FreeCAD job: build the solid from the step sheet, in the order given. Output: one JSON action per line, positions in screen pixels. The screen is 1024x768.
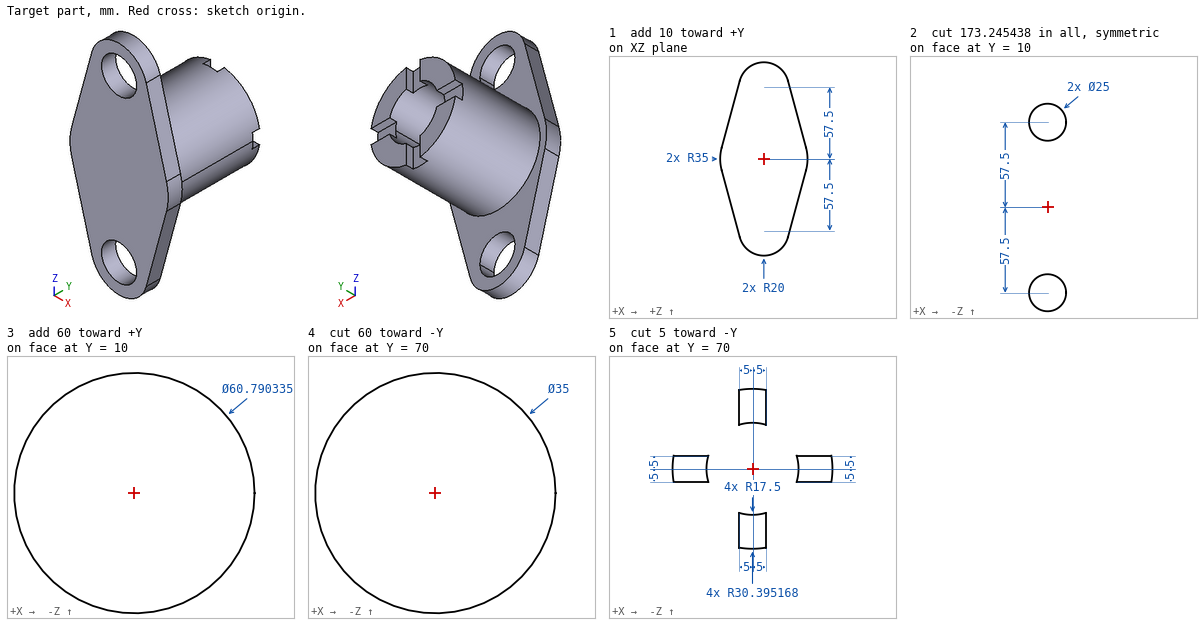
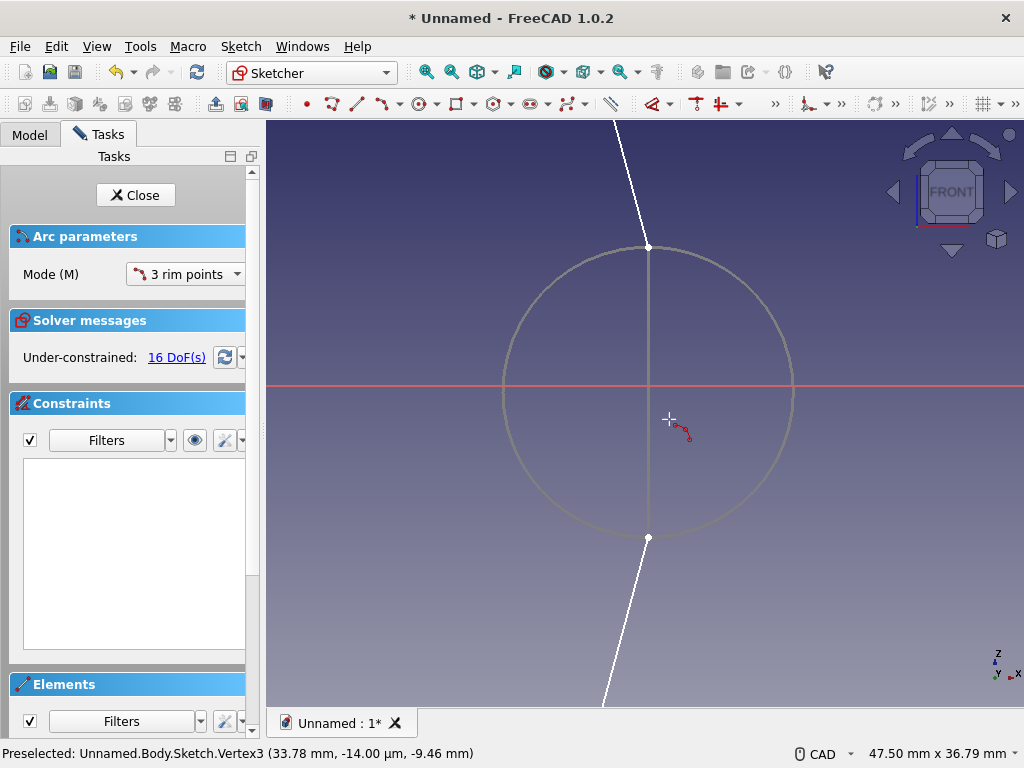
{"action": "left_click", "coordinate": [667, 416]}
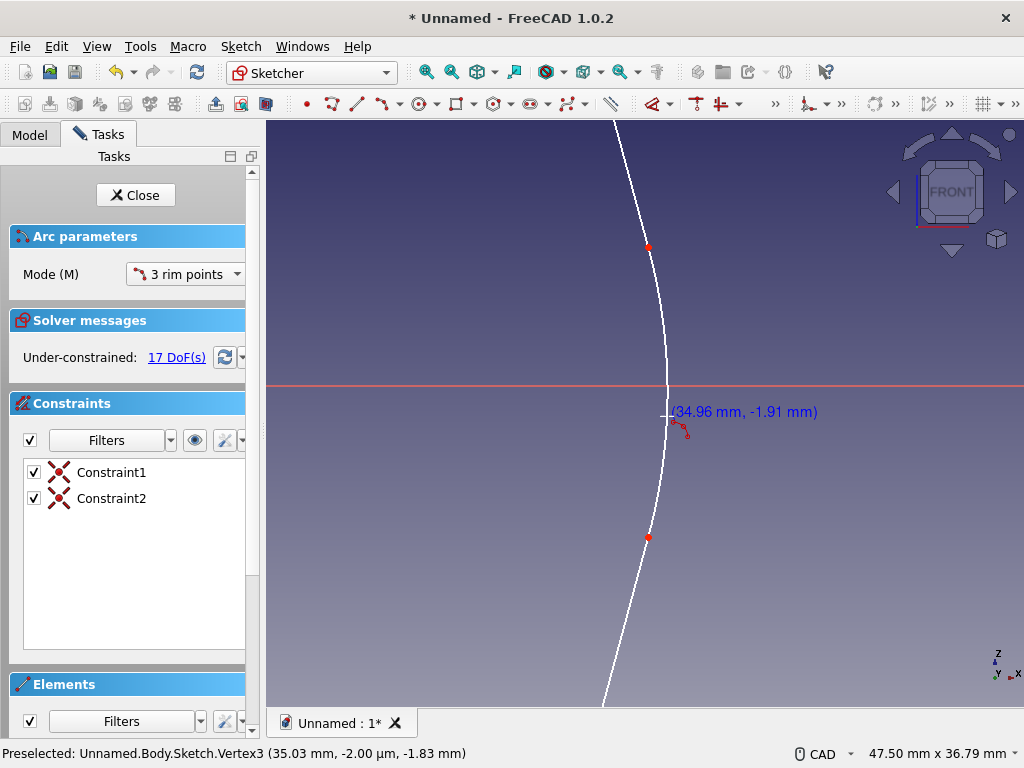
{"action": "scroll", "coordinate": [669, 419], "scroll_direction": "down", "scroll_amount": 9}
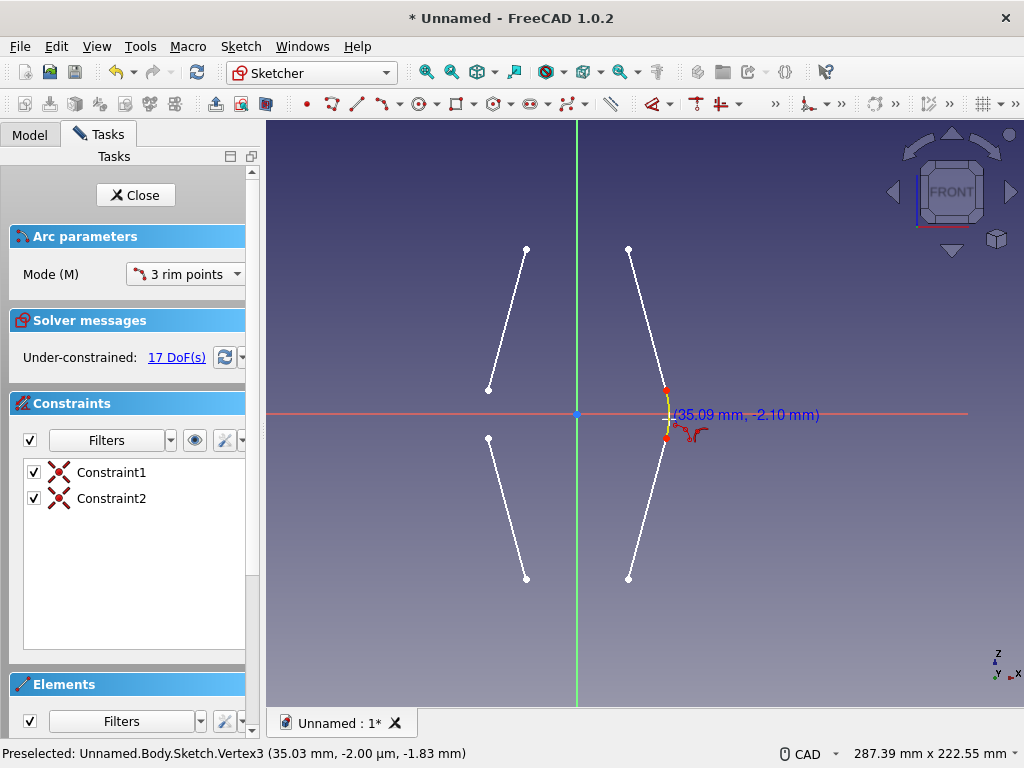
{"action": "left_click", "coordinate": [628, 580]}
{"action": "left_click", "coordinate": [526, 580]}
{"action": "left_click", "coordinate": [551, 611]}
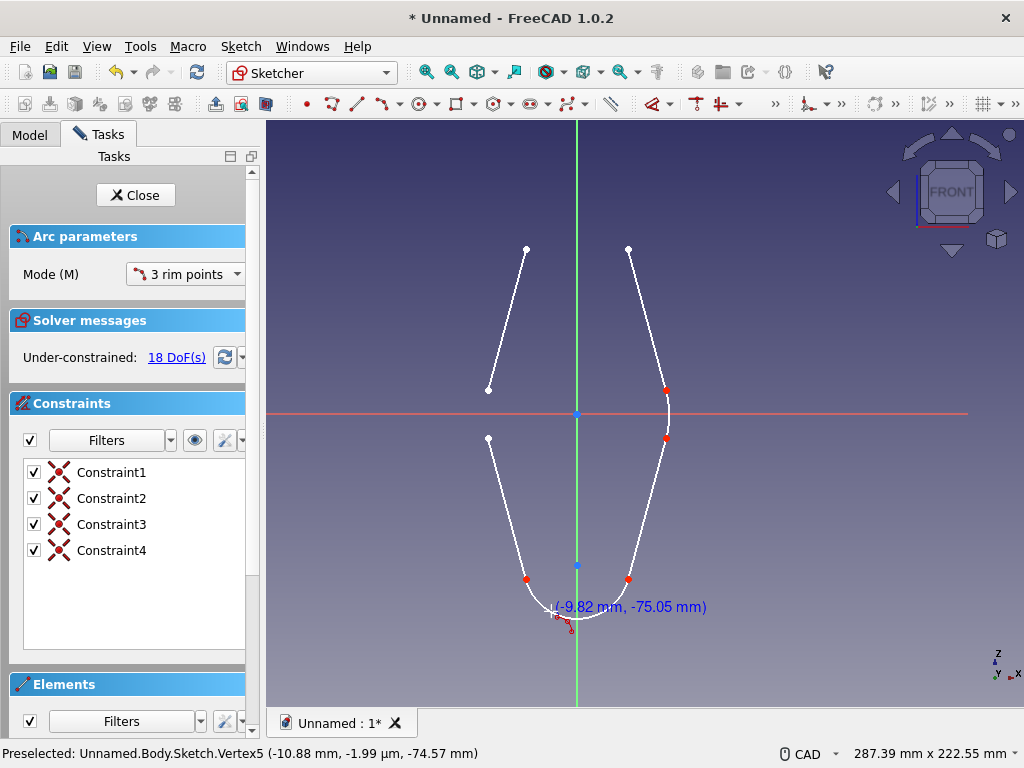
{"action": "left_click", "coordinate": [488, 439]}
{"action": "left_click", "coordinate": [488, 391]}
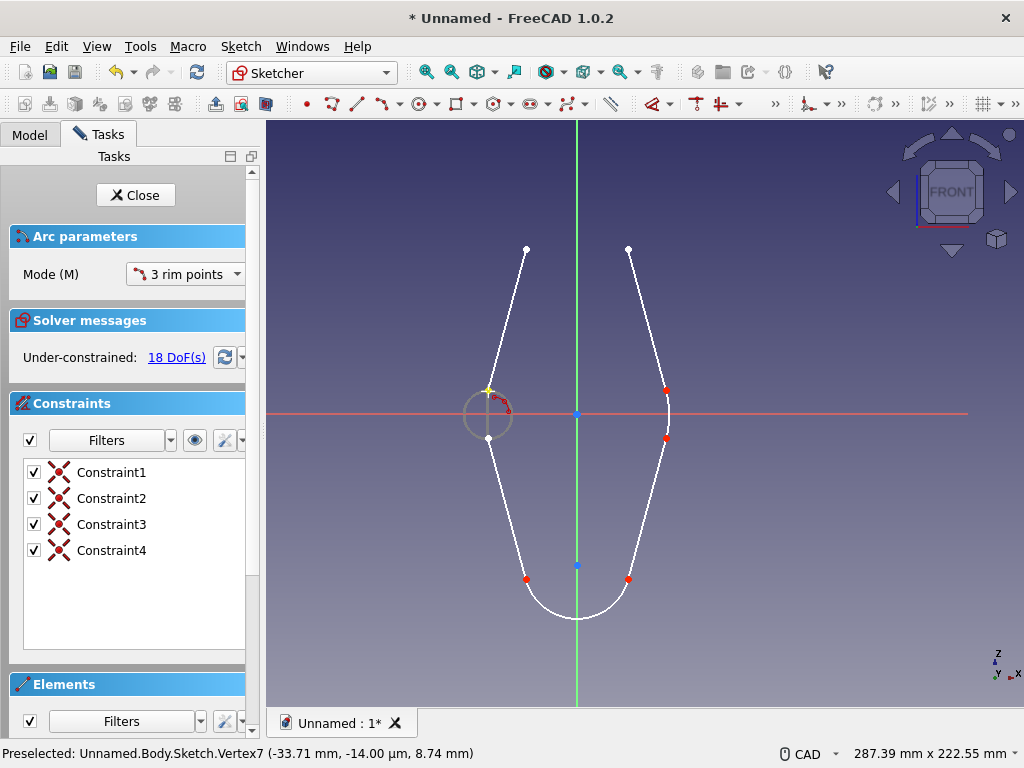
{"action": "scroll", "coordinate": [485, 409], "scroll_direction": "up", "scroll_amount": 9}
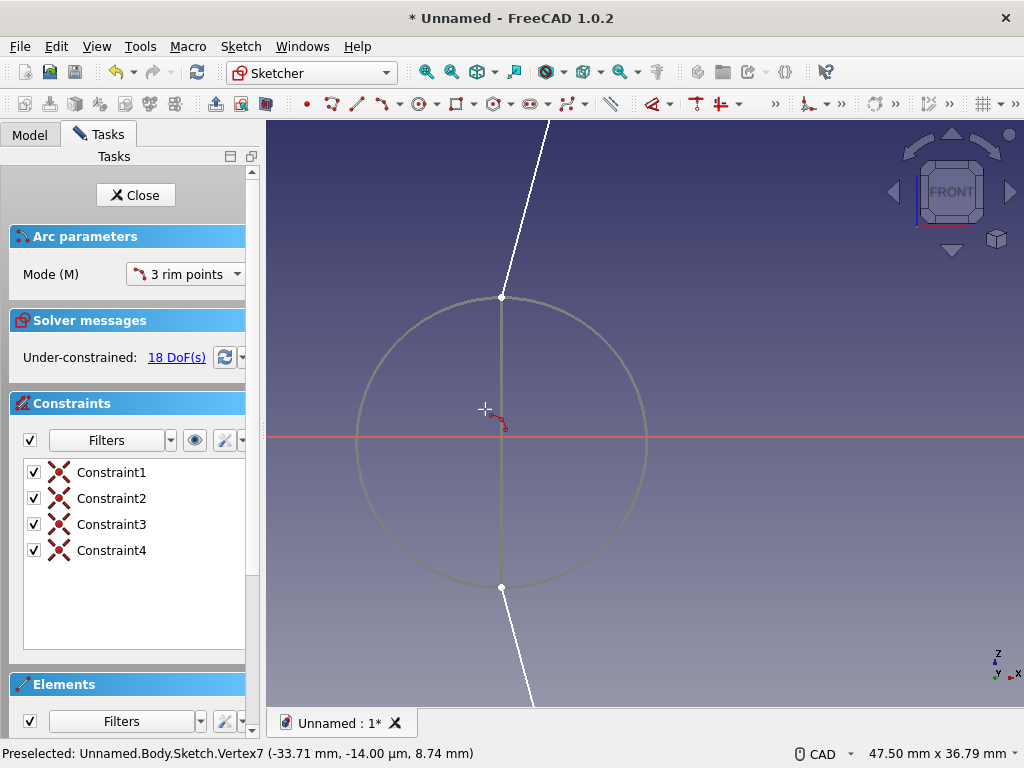
{"action": "left_click", "coordinate": [482, 408]}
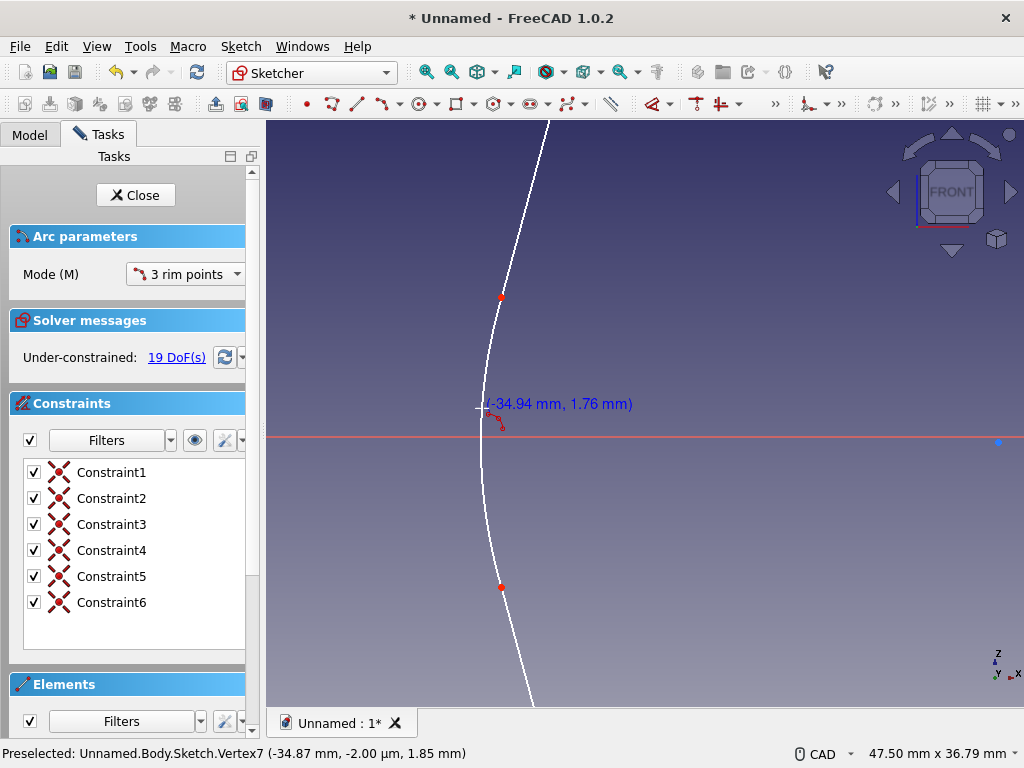
{"action": "scroll", "coordinate": [485, 409], "scroll_direction": "down", "scroll_amount": 9}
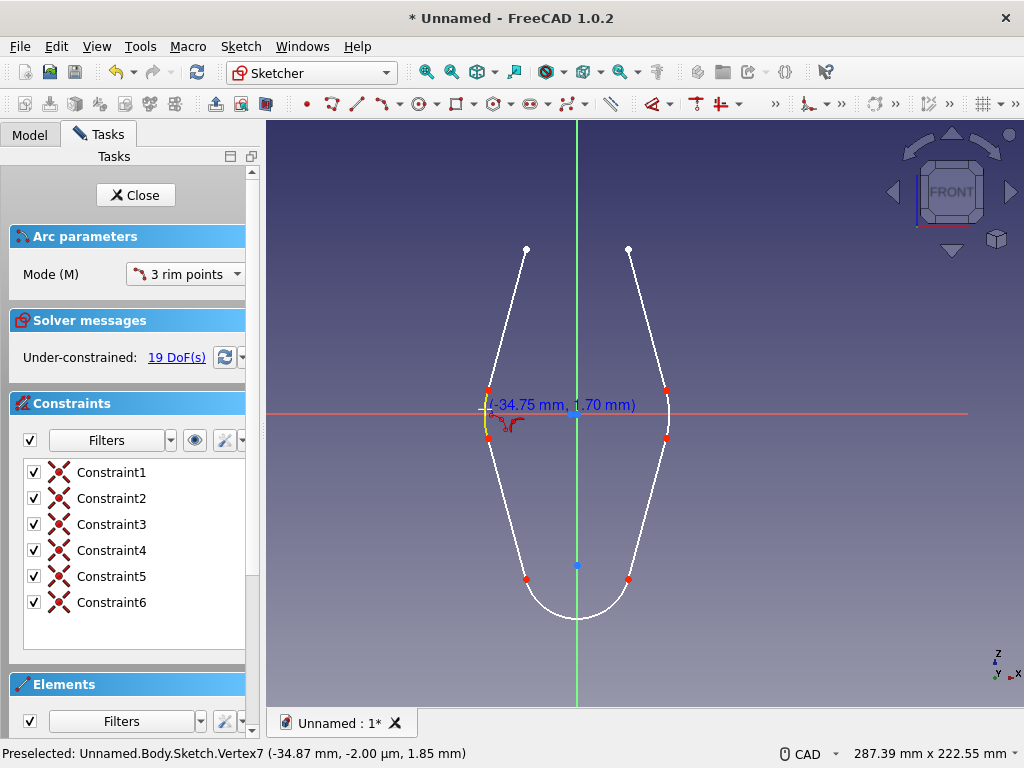
{"action": "left_click", "coordinate": [526, 250]}
{"action": "left_click", "coordinate": [628, 250]}
{"action": "left_click", "coordinate": [603, 217]}
{"action": "key", "text": "Escape"}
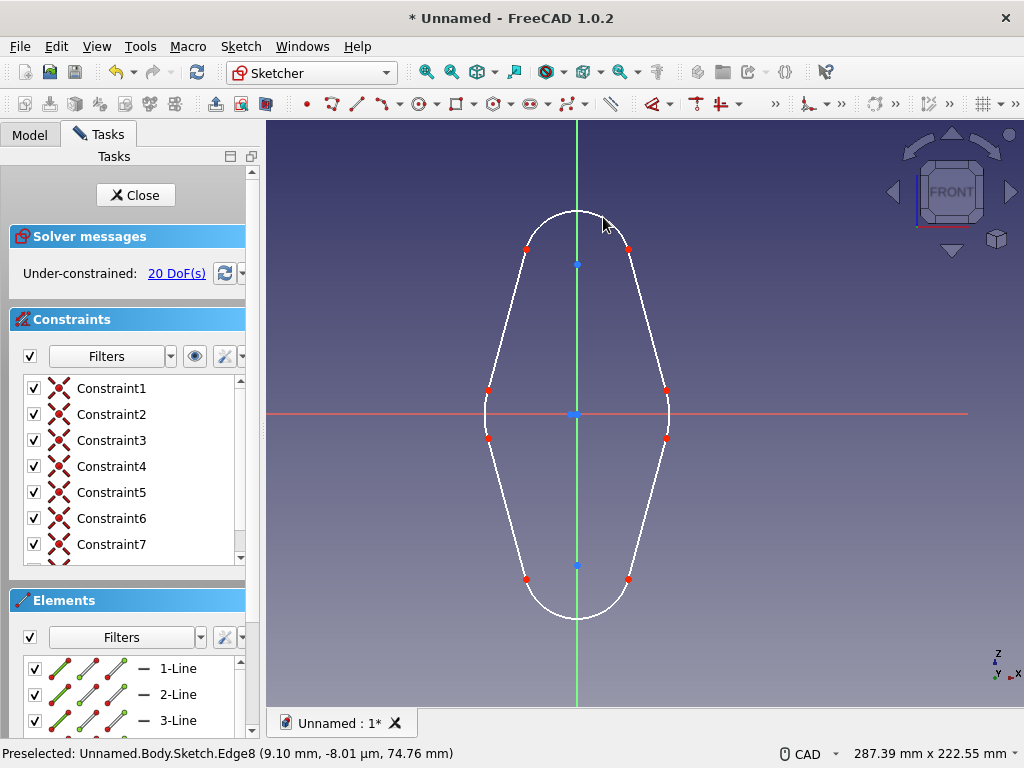
{"action": "left_click", "coordinate": [639, 292]}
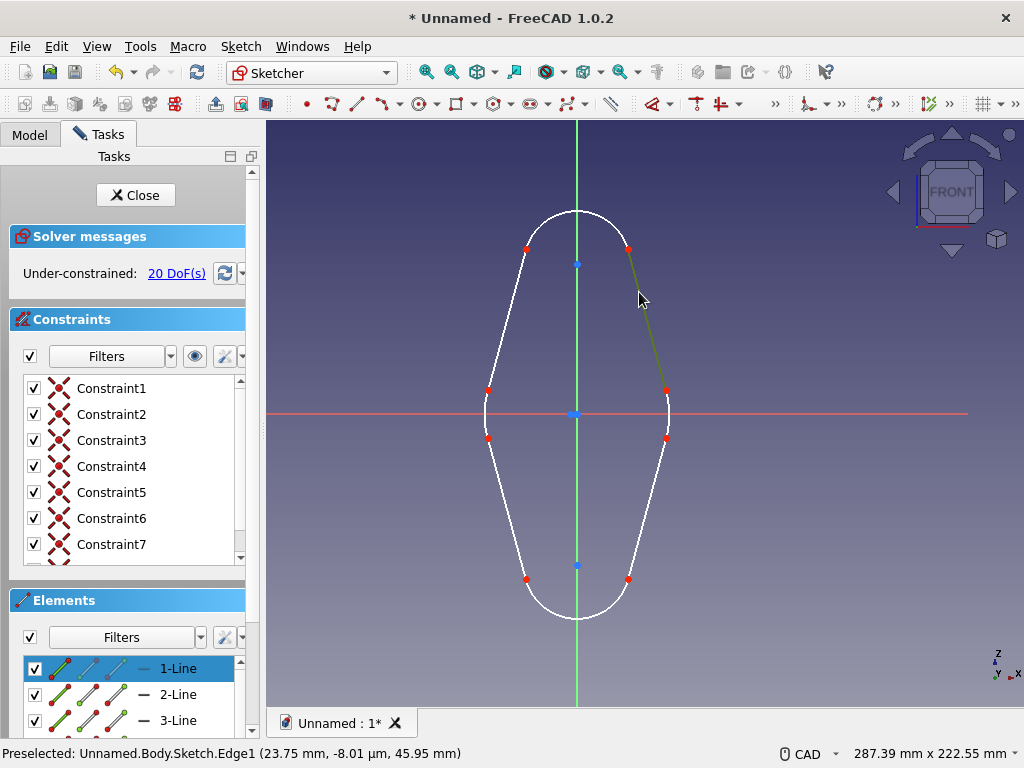
{"action": "scroll", "coordinate": [669, 425], "scroll_direction": "up", "scroll_amount": 2}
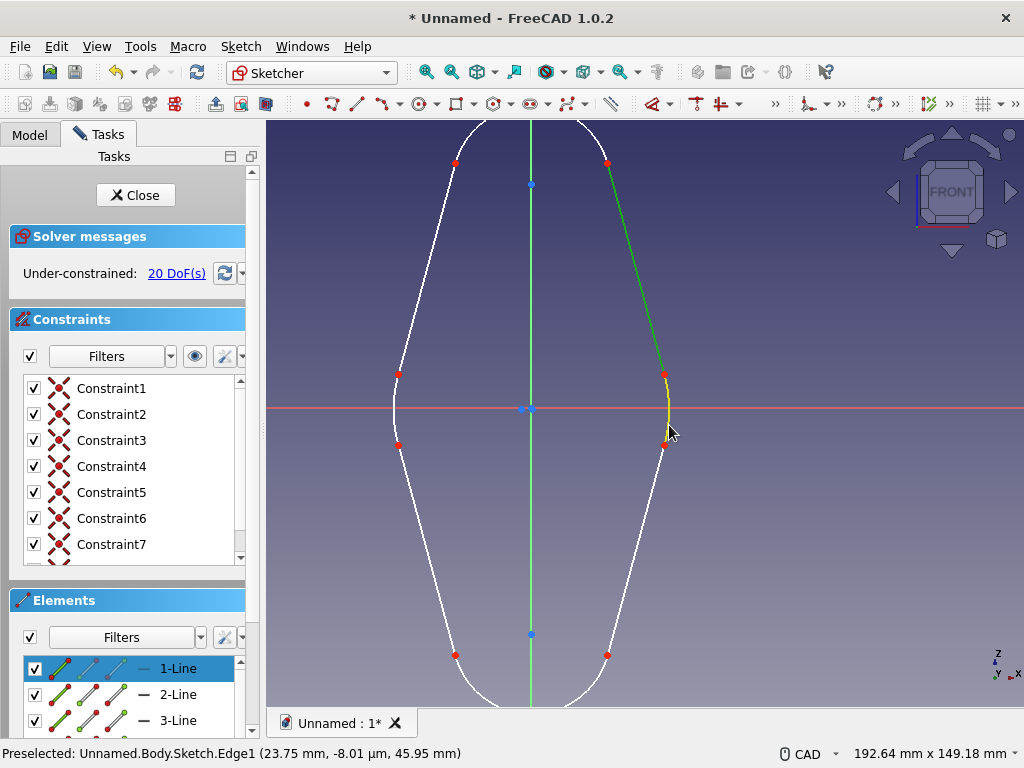
{"action": "left_click", "coordinate": [668, 424]}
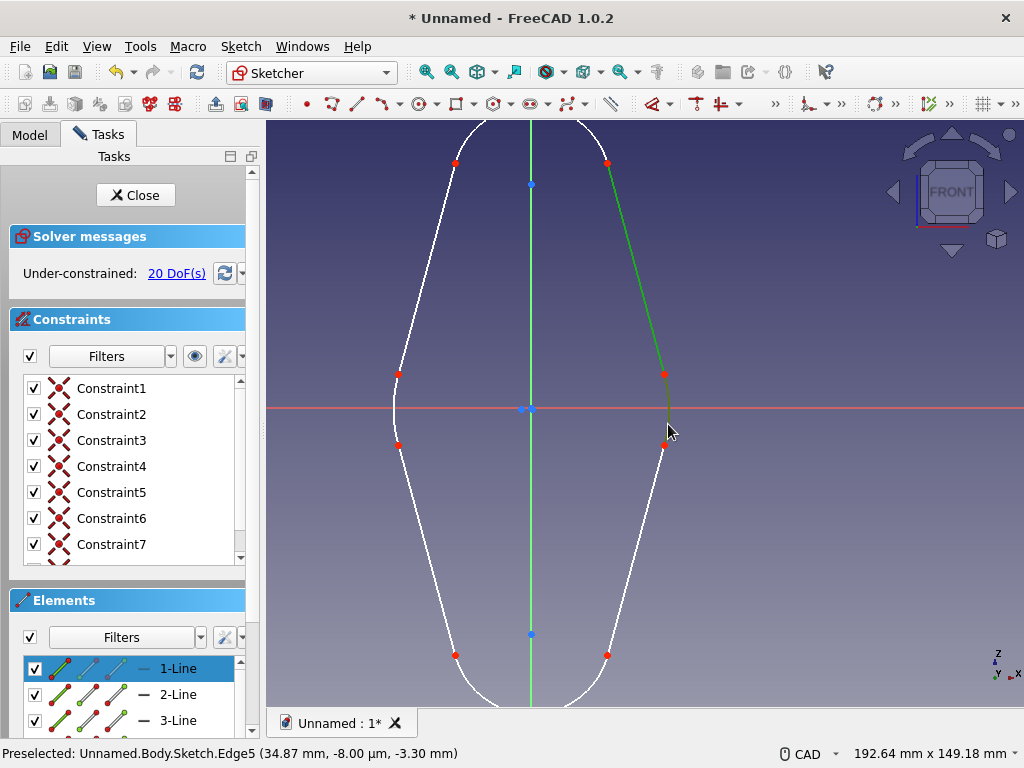
{"action": "key", "text": "t"}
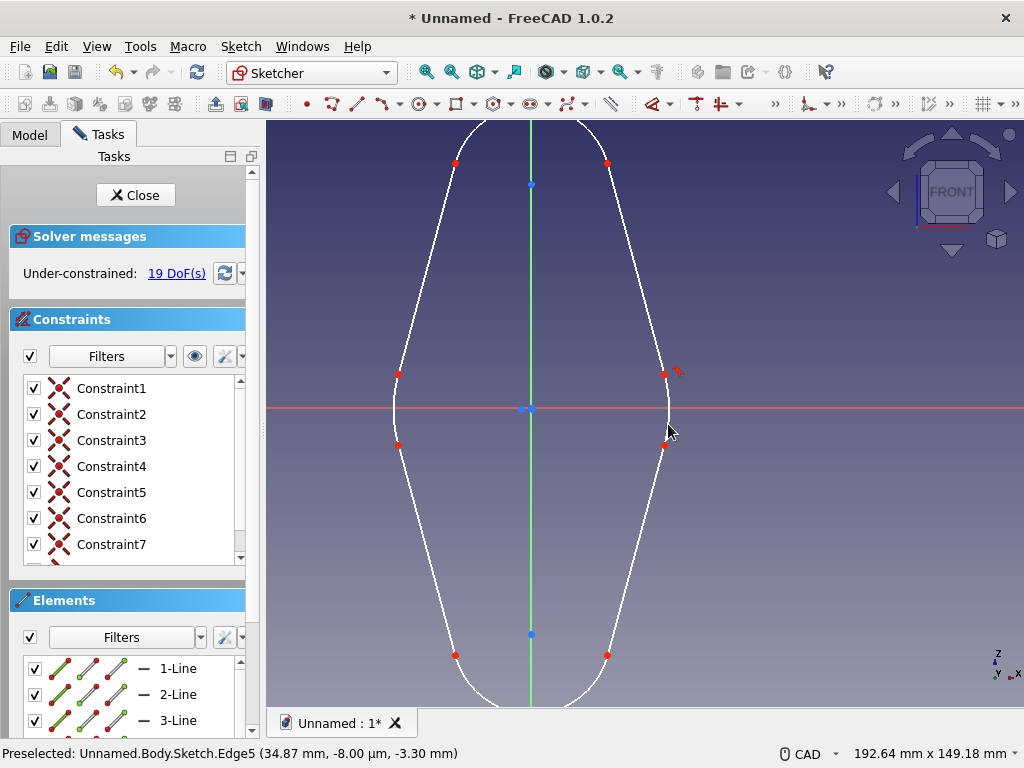
{"action": "left_click", "coordinate": [625, 227]}